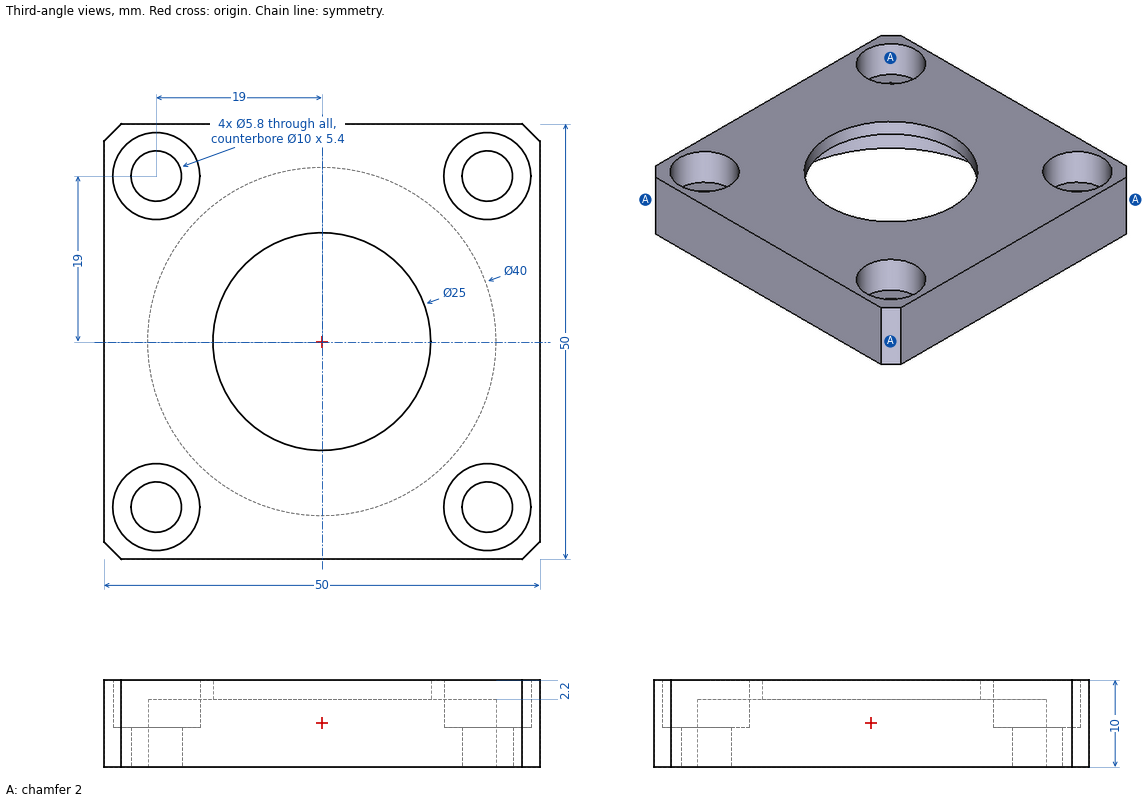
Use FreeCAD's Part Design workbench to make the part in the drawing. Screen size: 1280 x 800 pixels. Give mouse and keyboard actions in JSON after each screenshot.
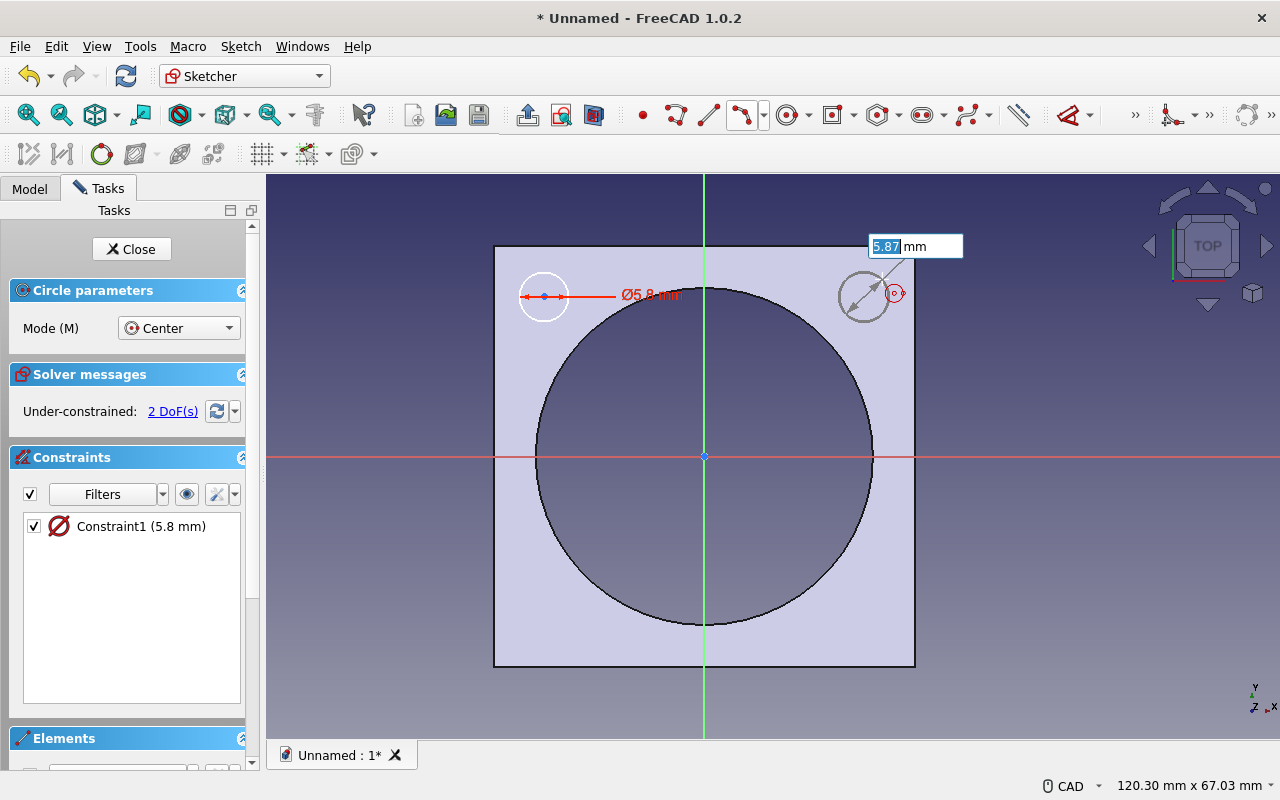
{"action": "type", "text": "5.8"}
{"action": "key", "text": "Return"}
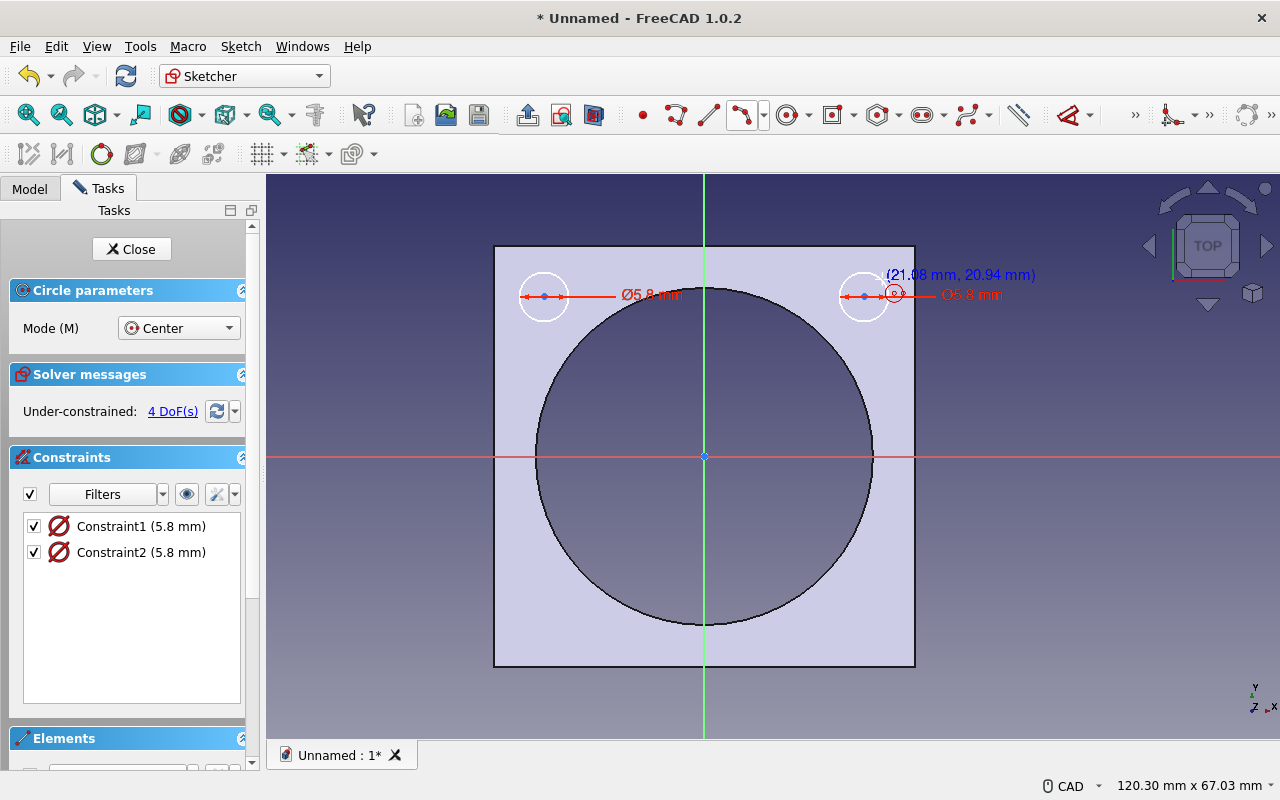
{"action": "left_click", "coordinate": [544, 617]}
{"action": "mouse_move", "coordinate": [561, 599]}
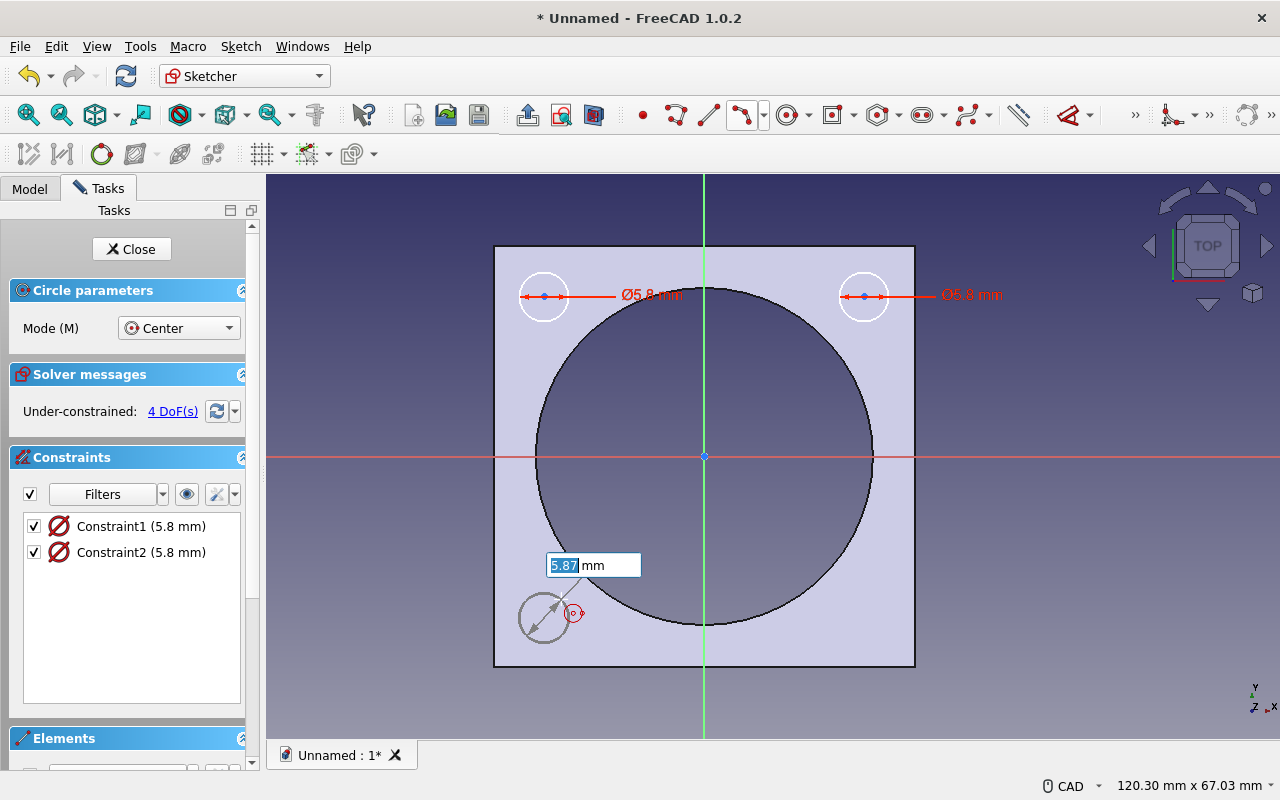
{"action": "type", "text": "5.8"}
{"action": "key", "text": "Return"}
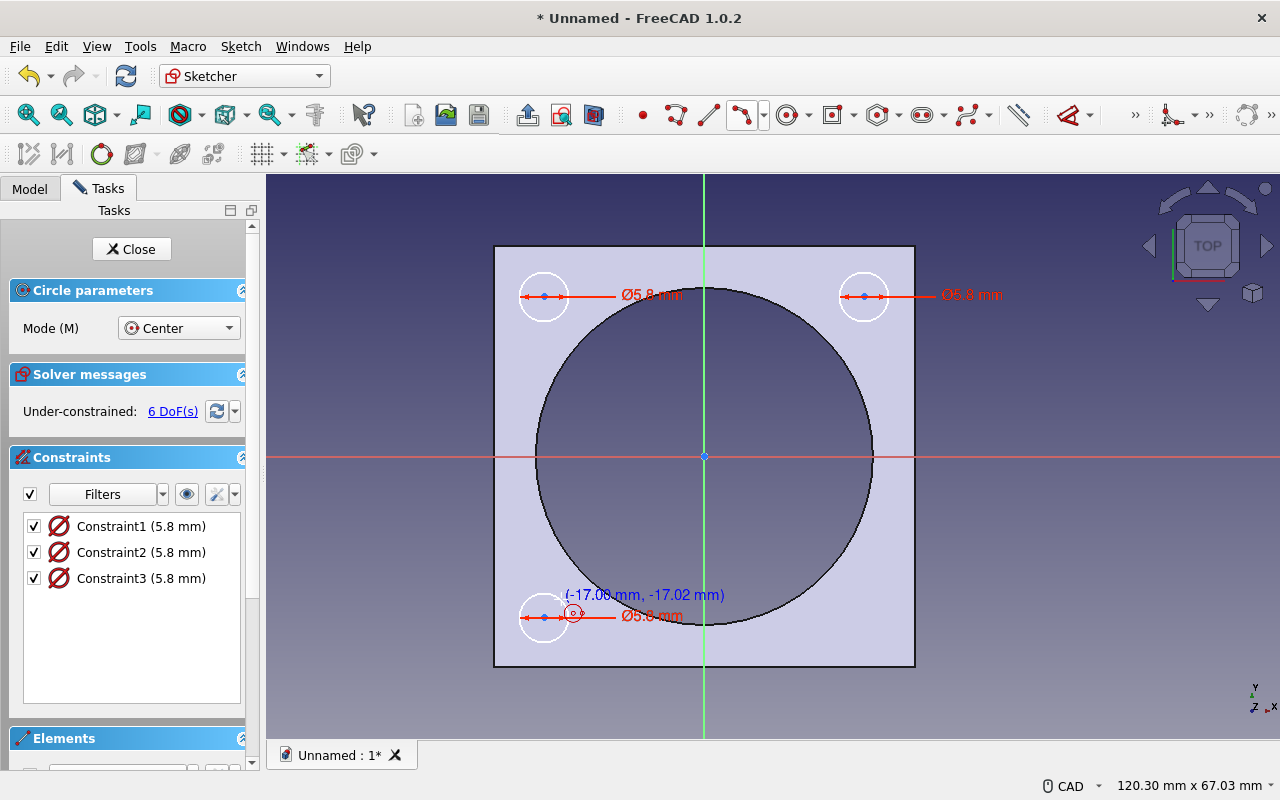
{"action": "left_click", "coordinate": [864, 617]}
{"action": "mouse_move", "coordinate": [882, 599]}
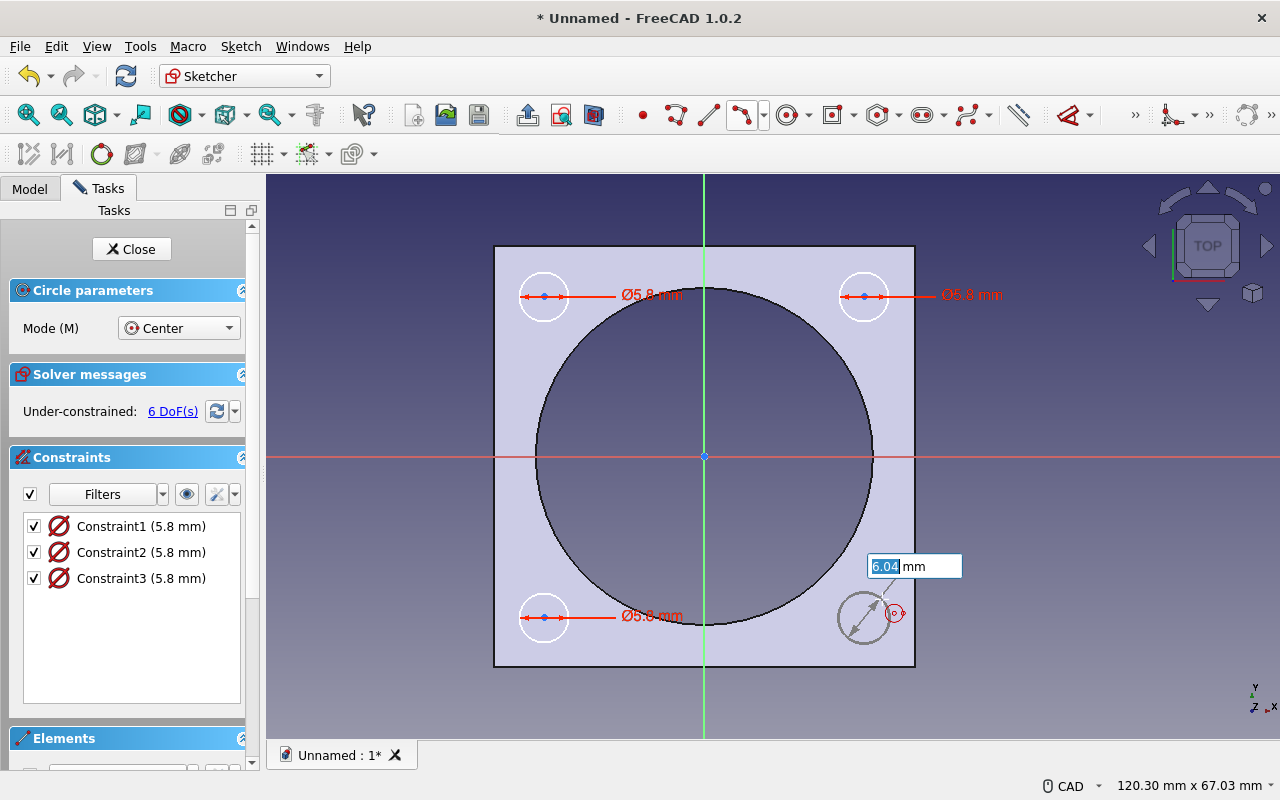
{"action": "type", "text": "5.8"}
{"action": "key", "text": "Return"}
{"action": "key", "text": "Escape"}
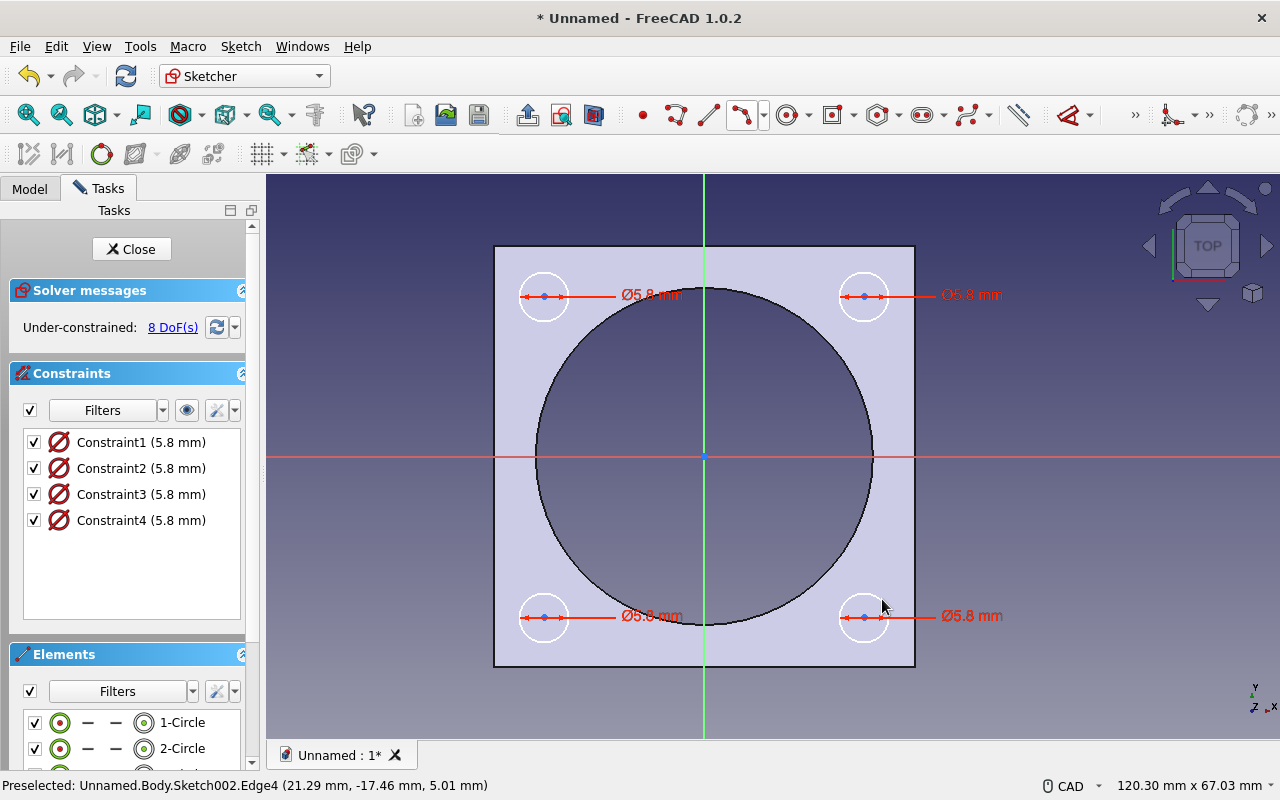
{"action": "left_click", "coordinate": [544, 297]}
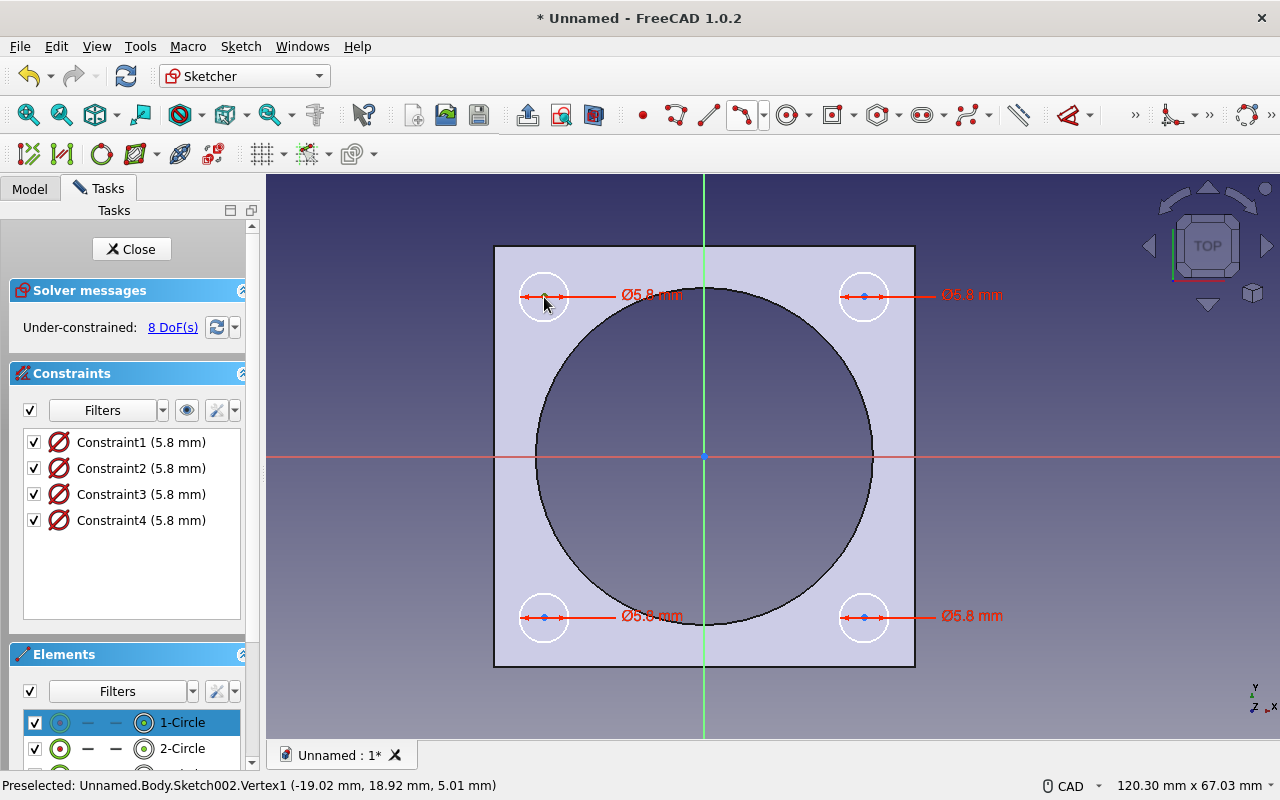
{"action": "left_click", "coordinate": [864, 297]}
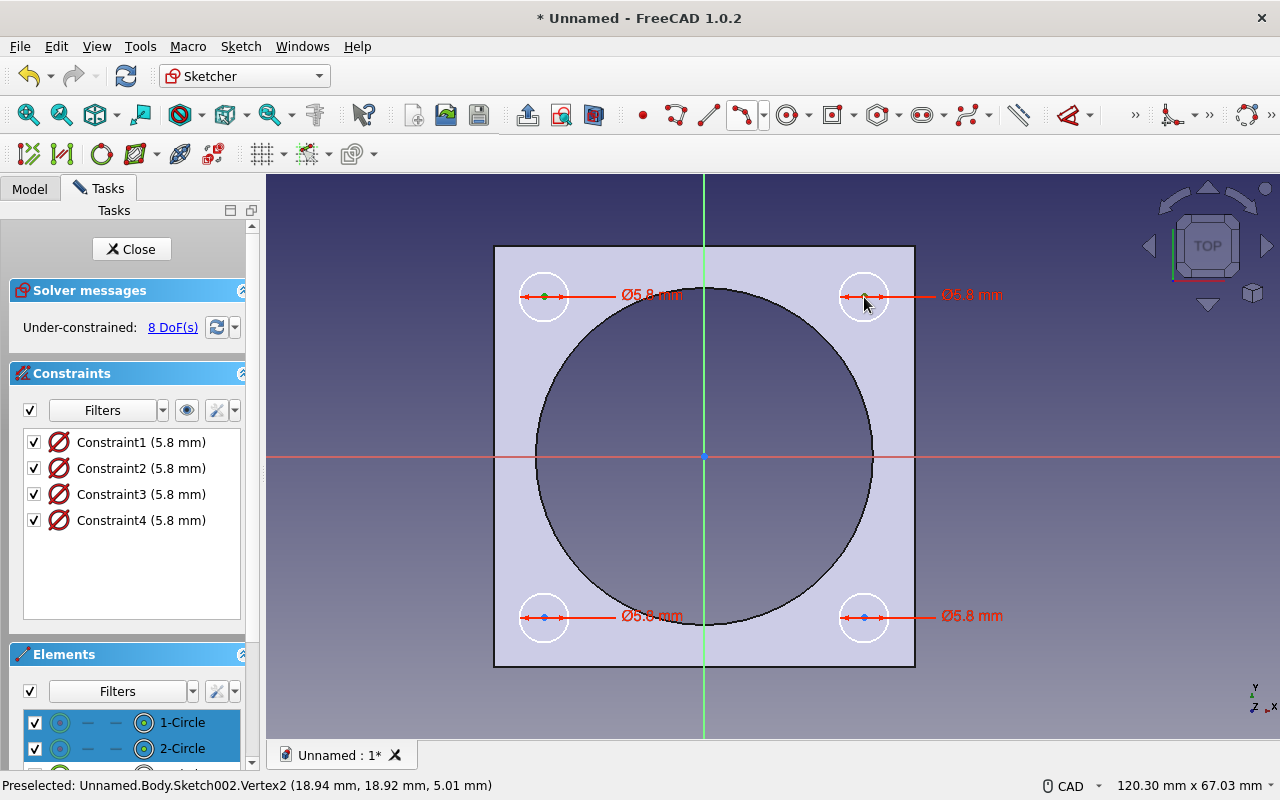
{"action": "left_click", "coordinate": [704, 675]}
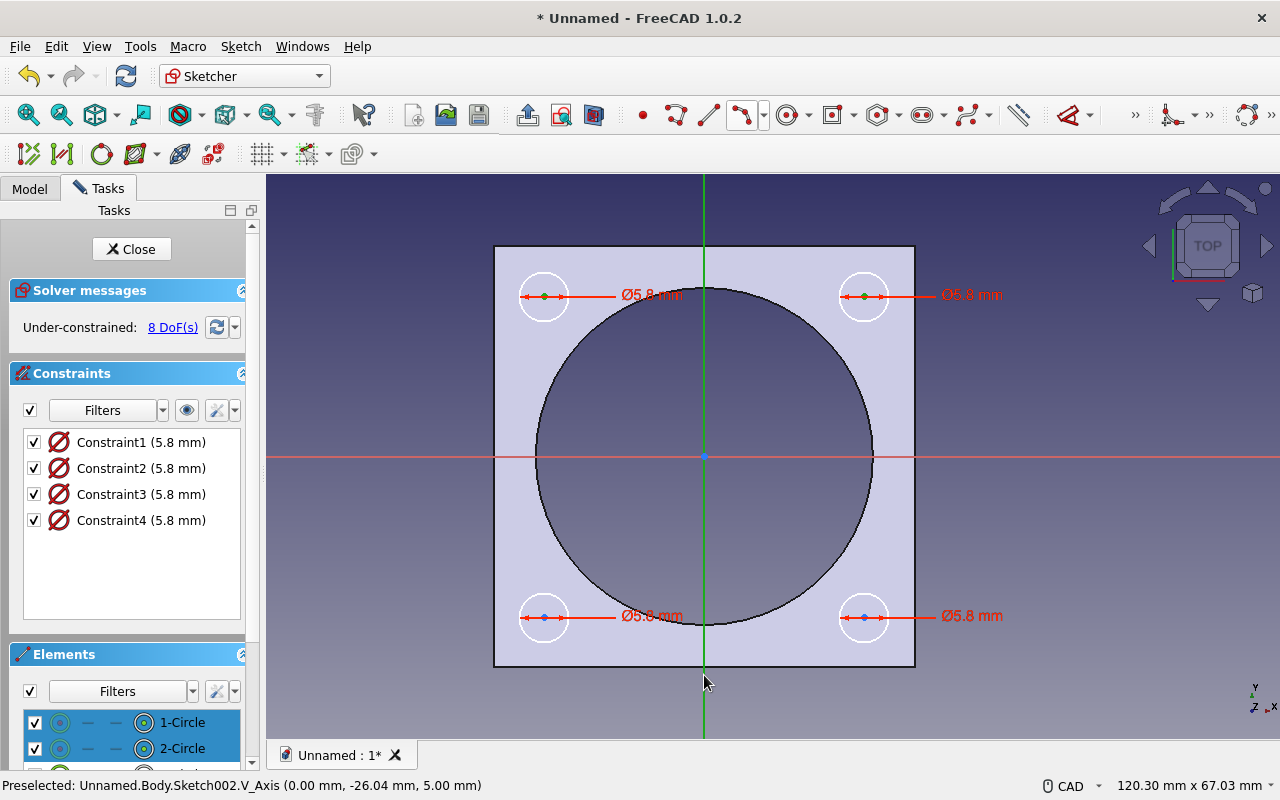
{"action": "key", "text": "s"}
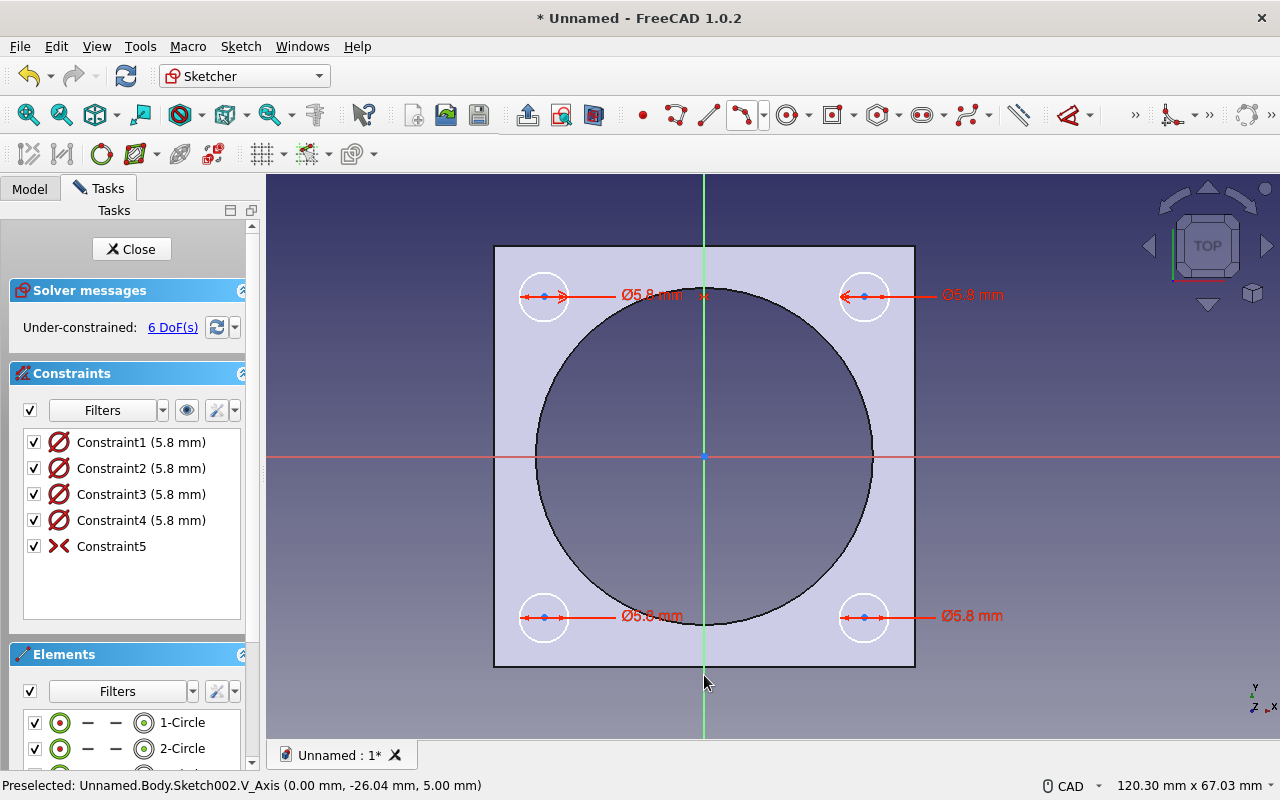
{"action": "left_click", "coordinate": [544, 297]}